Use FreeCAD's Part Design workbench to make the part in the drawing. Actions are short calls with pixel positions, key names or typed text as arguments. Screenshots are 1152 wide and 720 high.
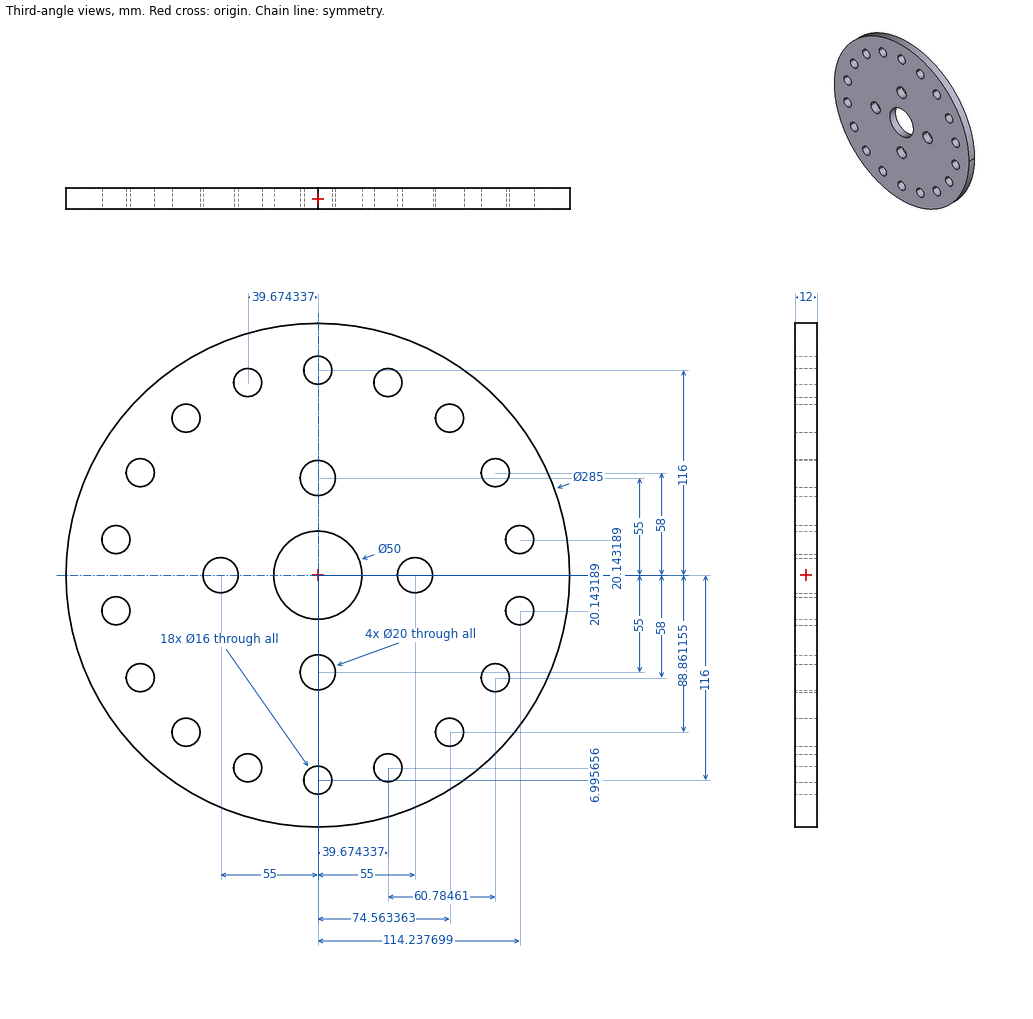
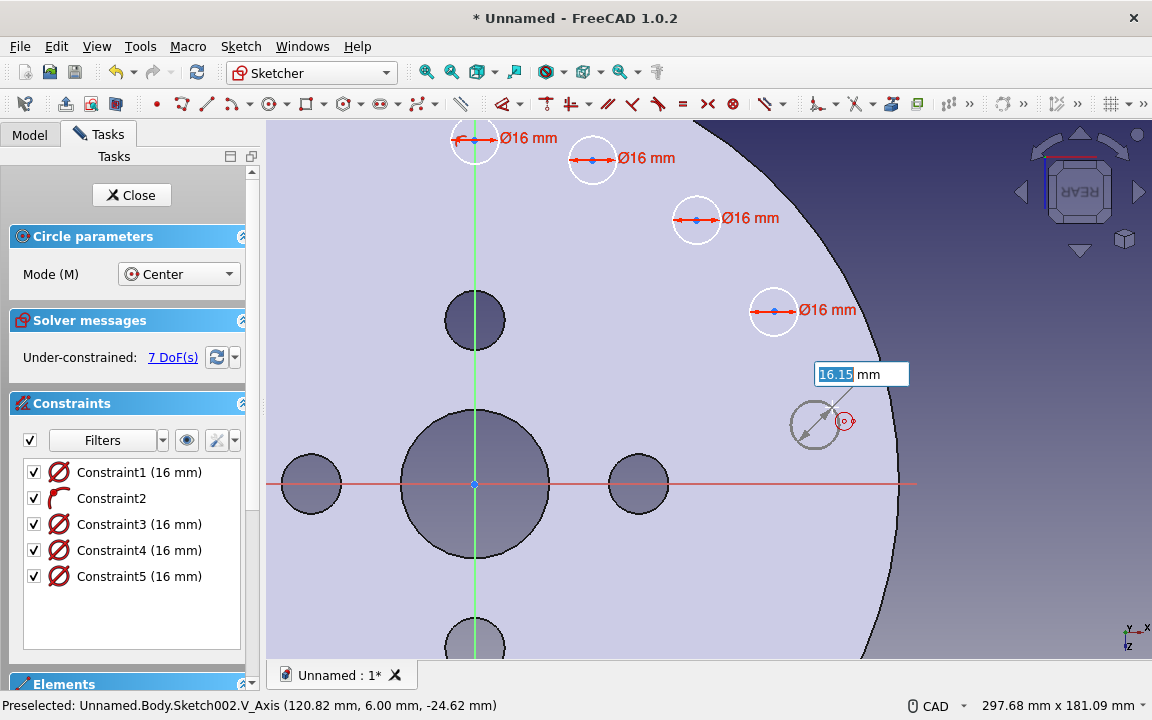
text(16)
key(Return)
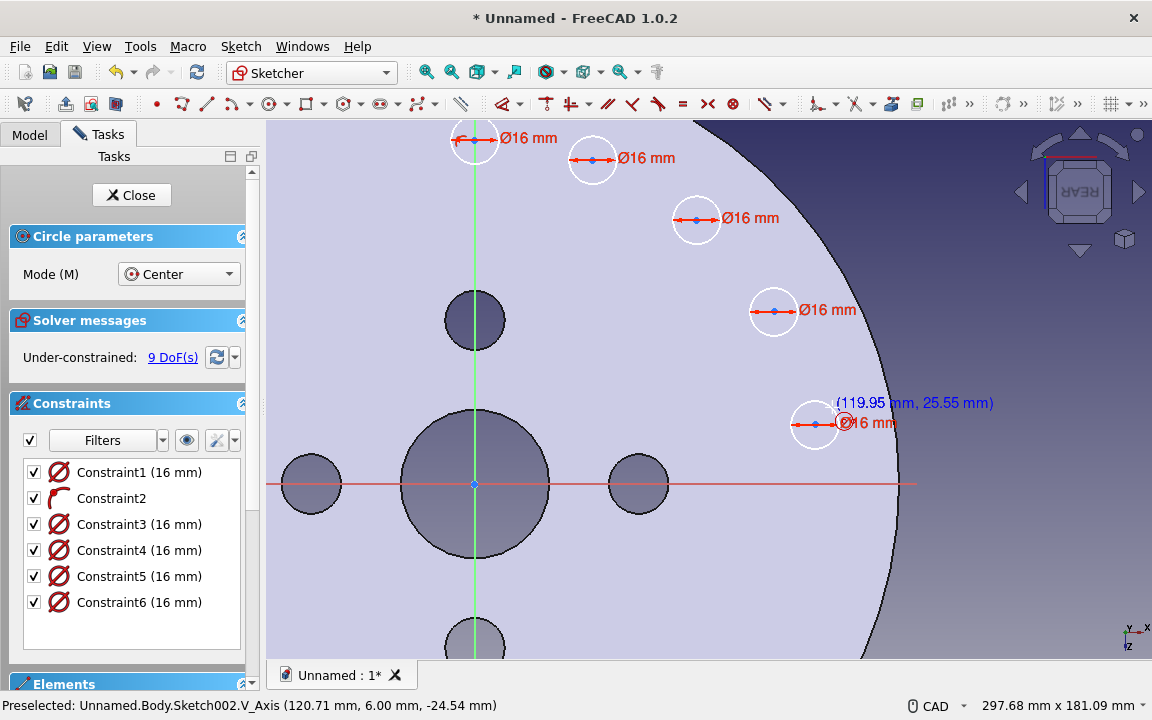
click(815, 544)
move(832, 527)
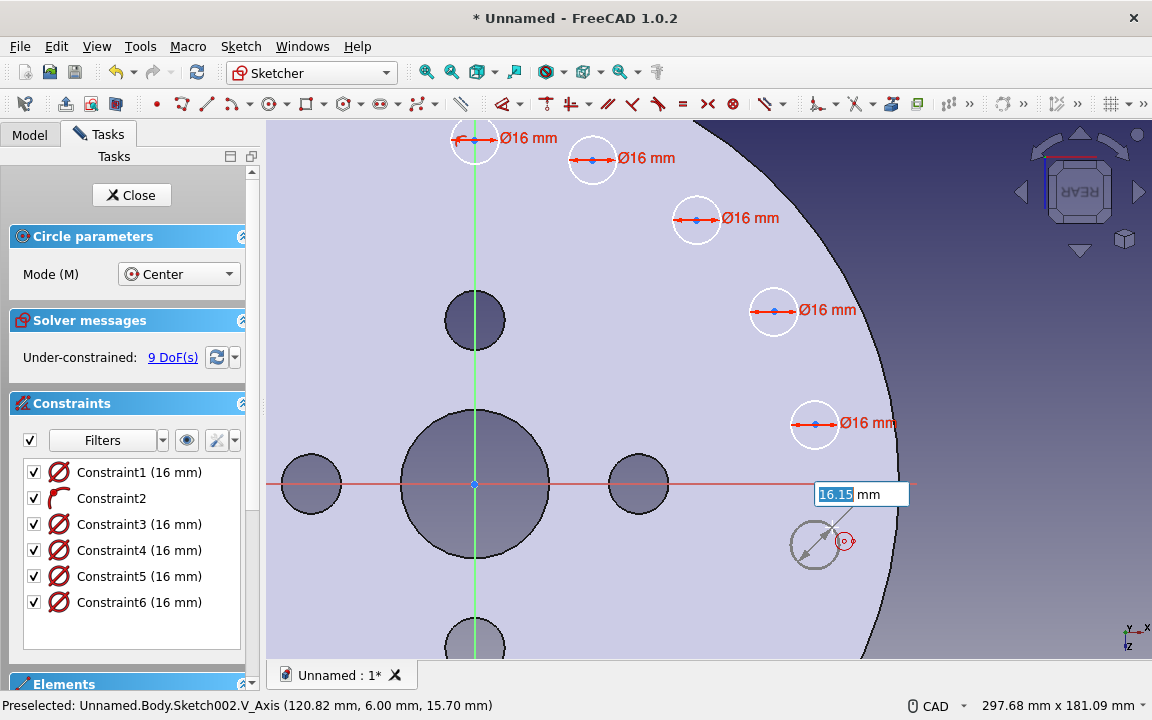
text(16)
key(Return)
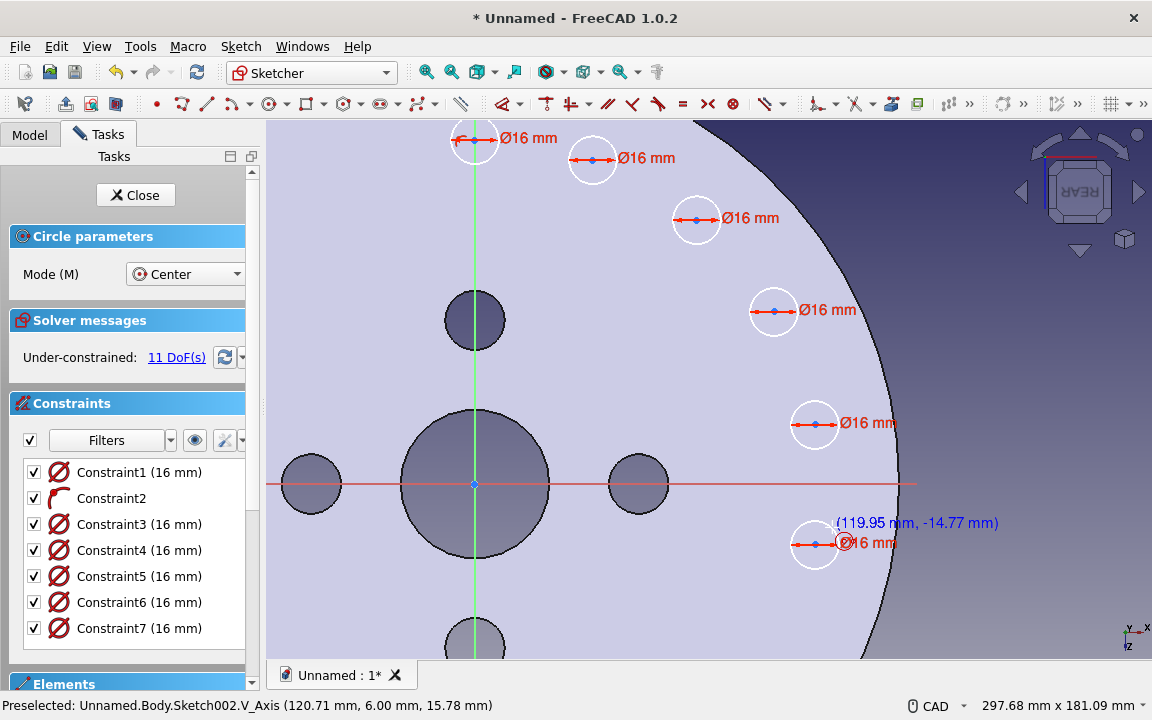
scroll(776, 312, down, 4)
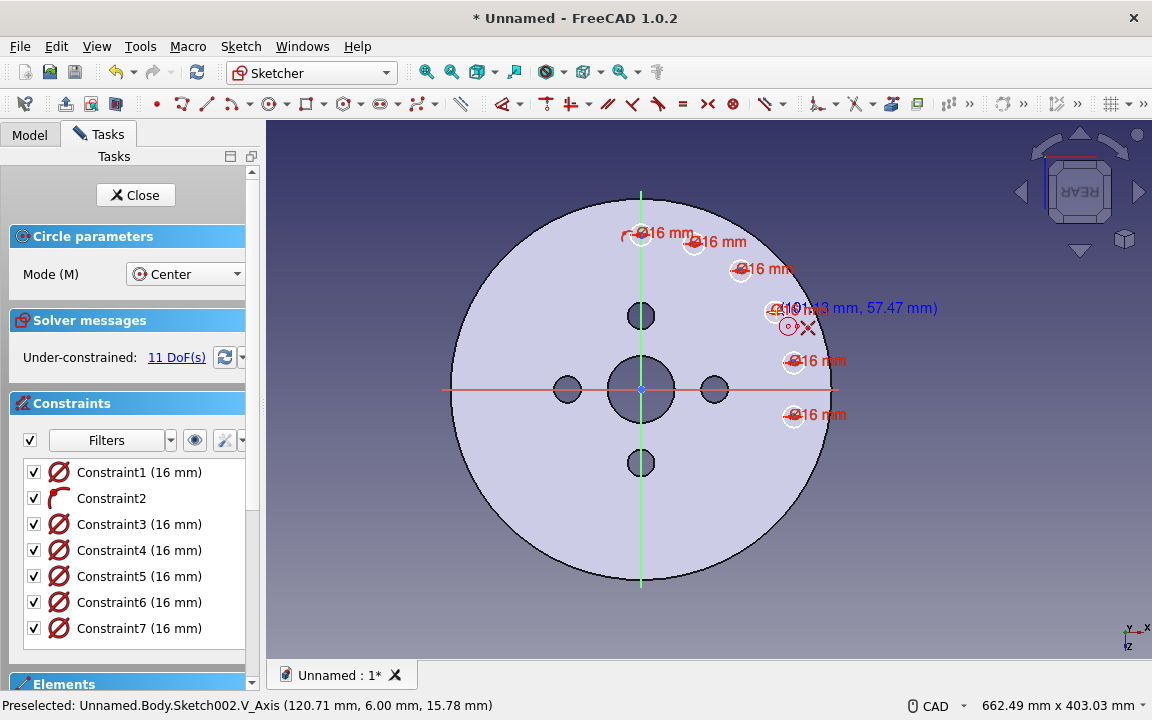
scroll(775, 467, up, 4)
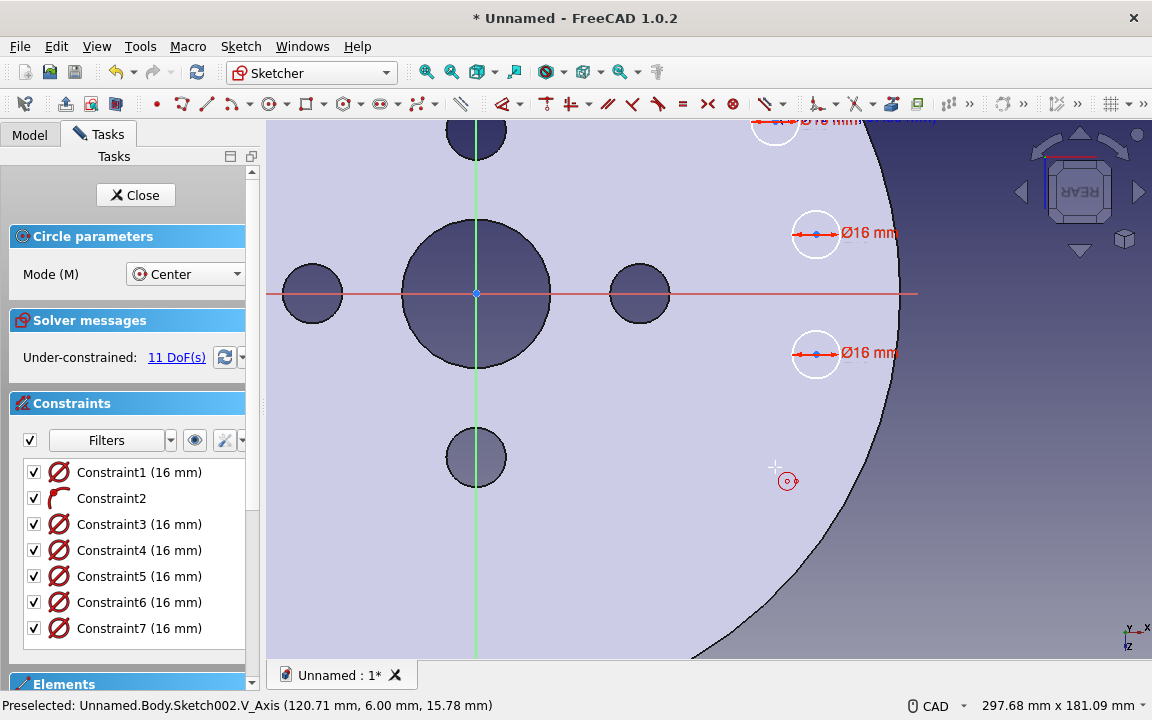
click(775, 466)
move(792, 450)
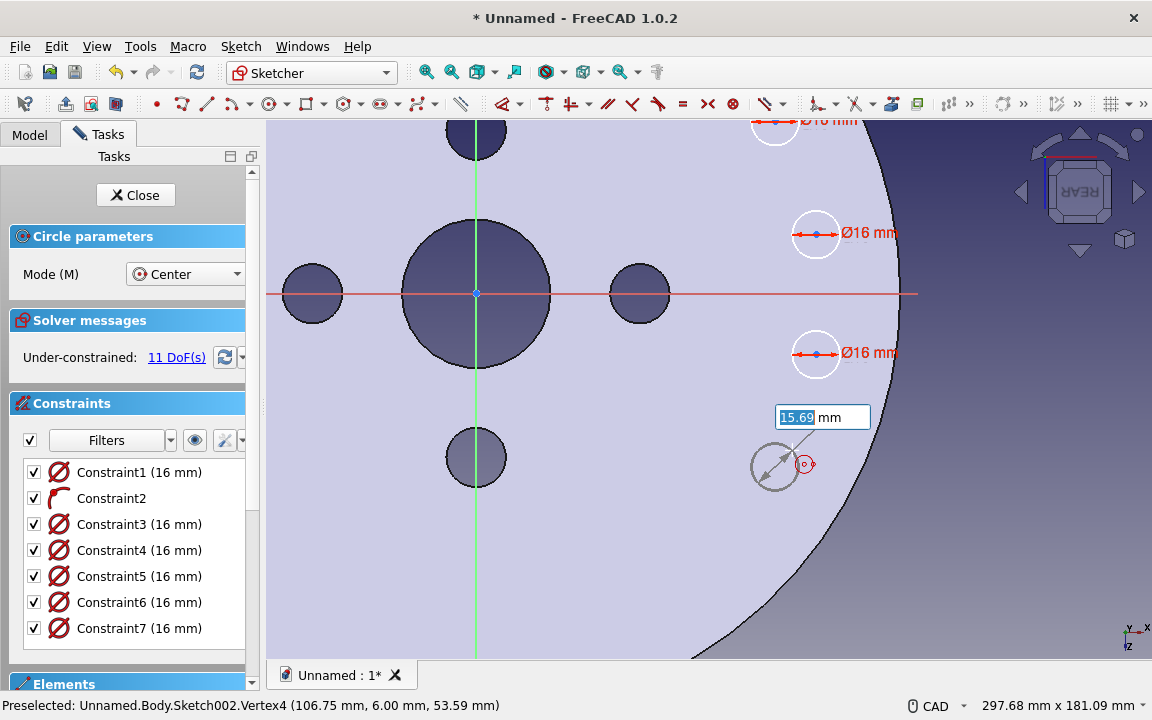
text(16)
key(Return)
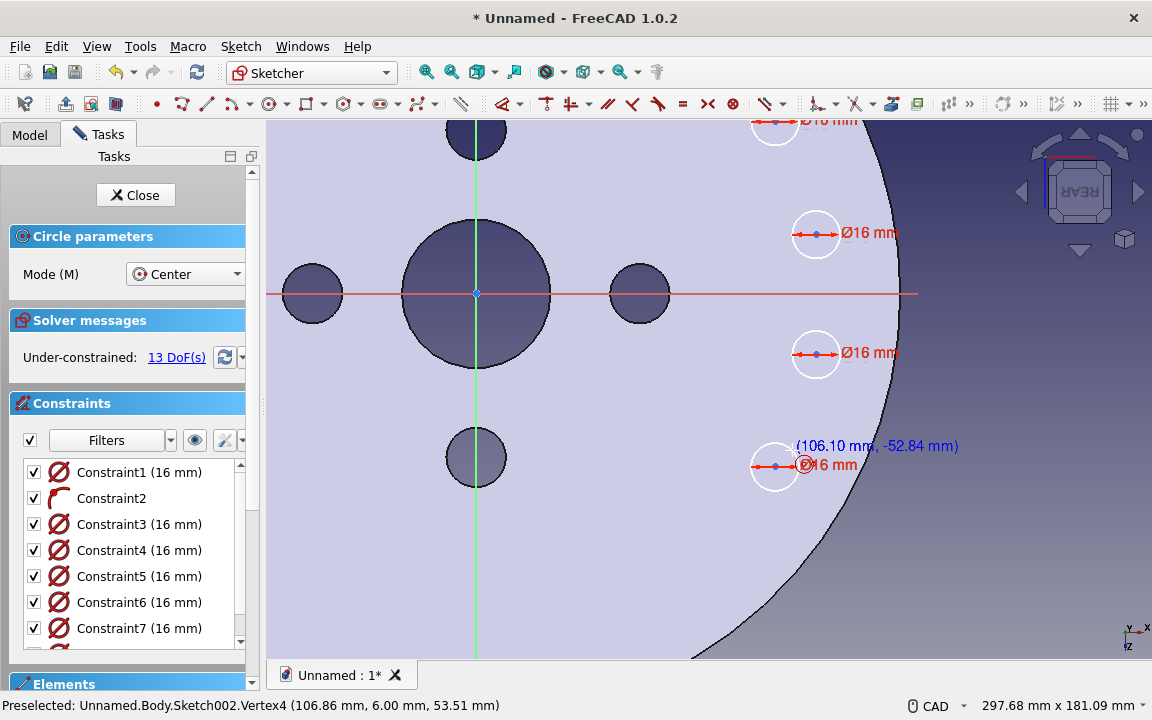
click(698, 558)
move(715, 541)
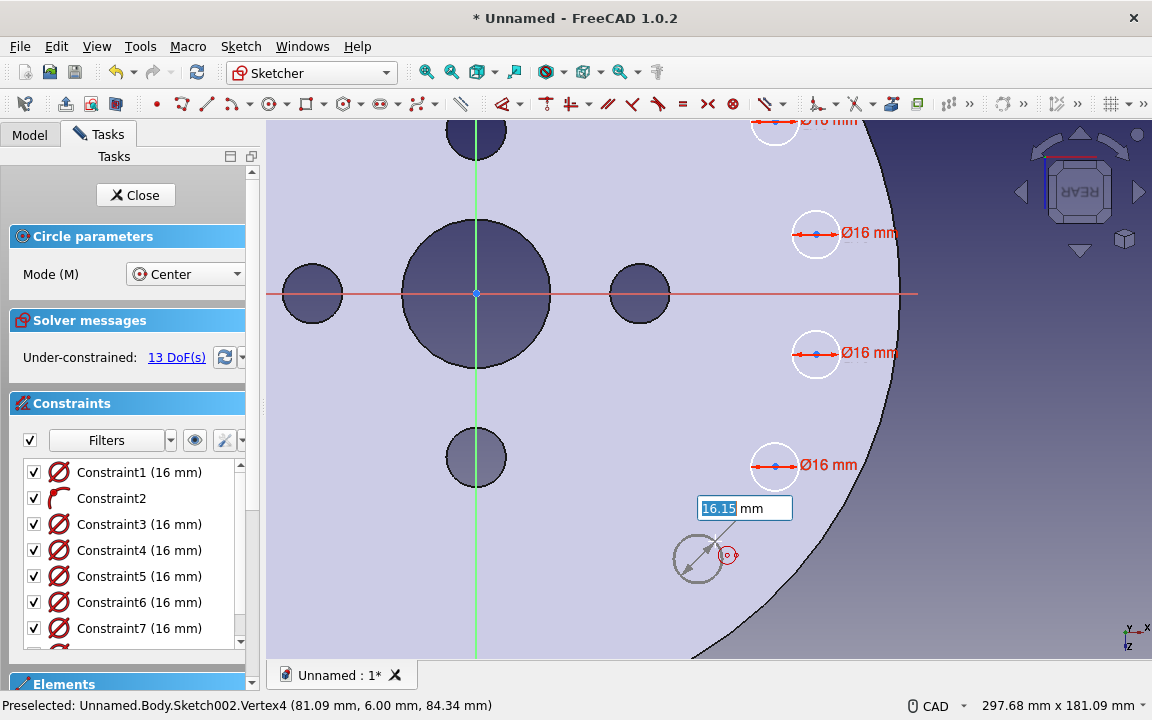
text(16)
key(Return)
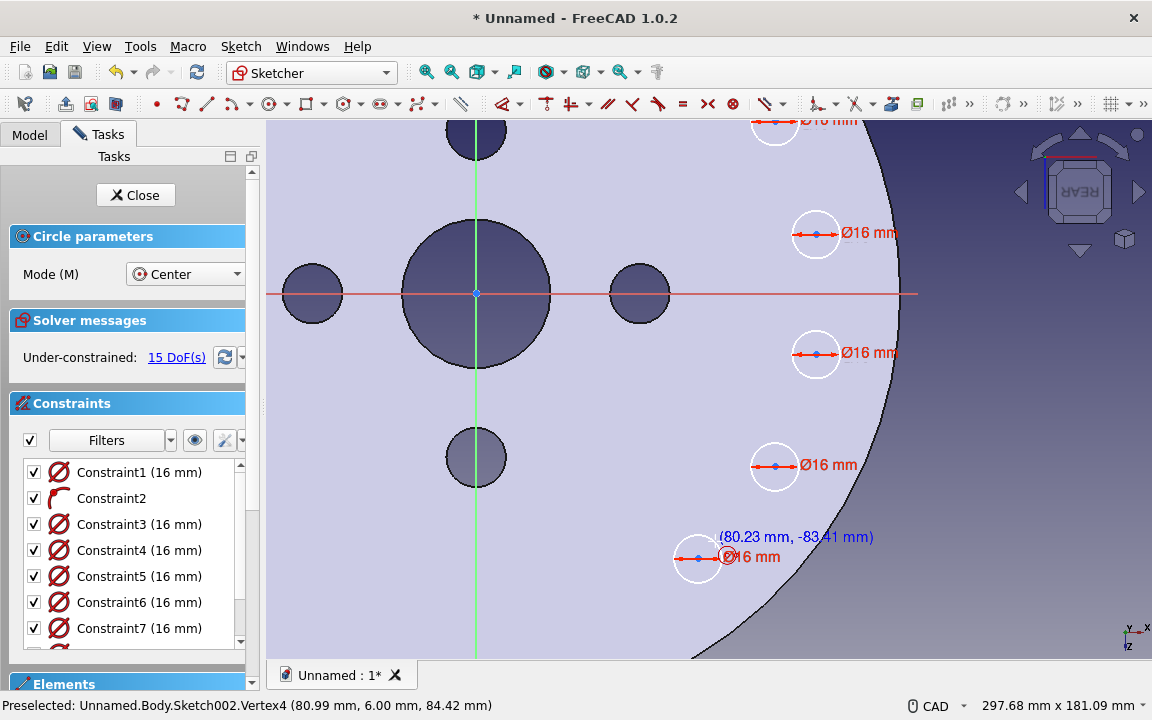
click(594, 618)
move(611, 601)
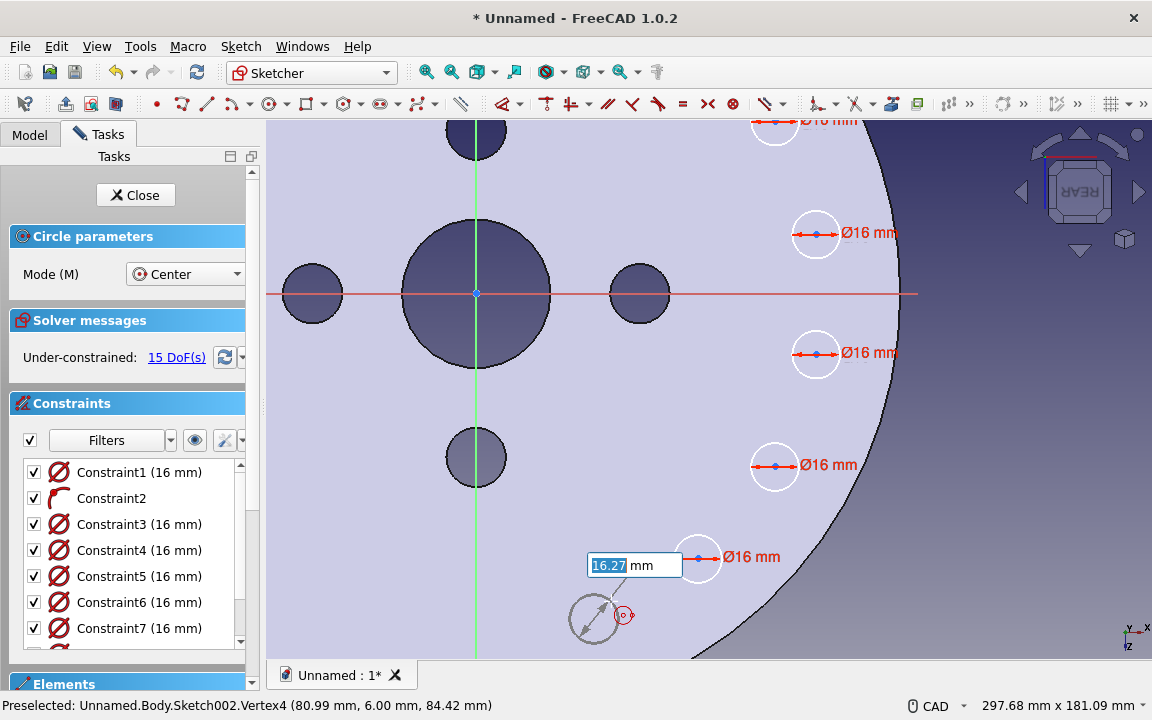
text(16)
key(Return)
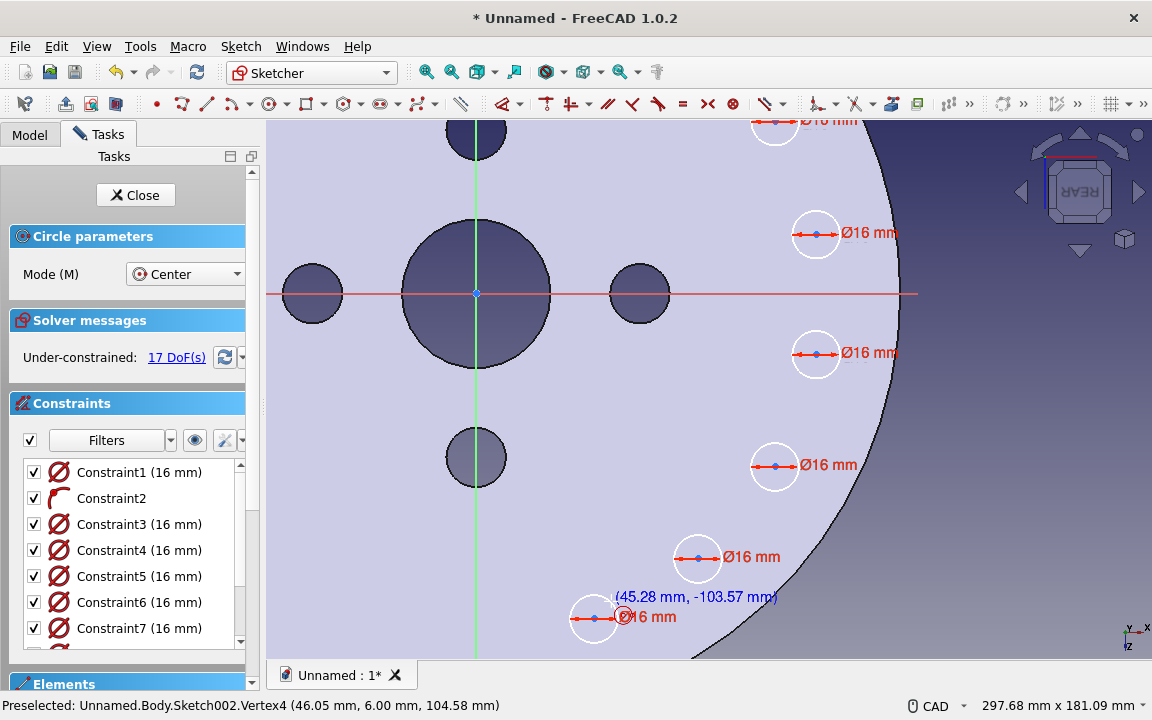
scroll(775, 468, down, 4)